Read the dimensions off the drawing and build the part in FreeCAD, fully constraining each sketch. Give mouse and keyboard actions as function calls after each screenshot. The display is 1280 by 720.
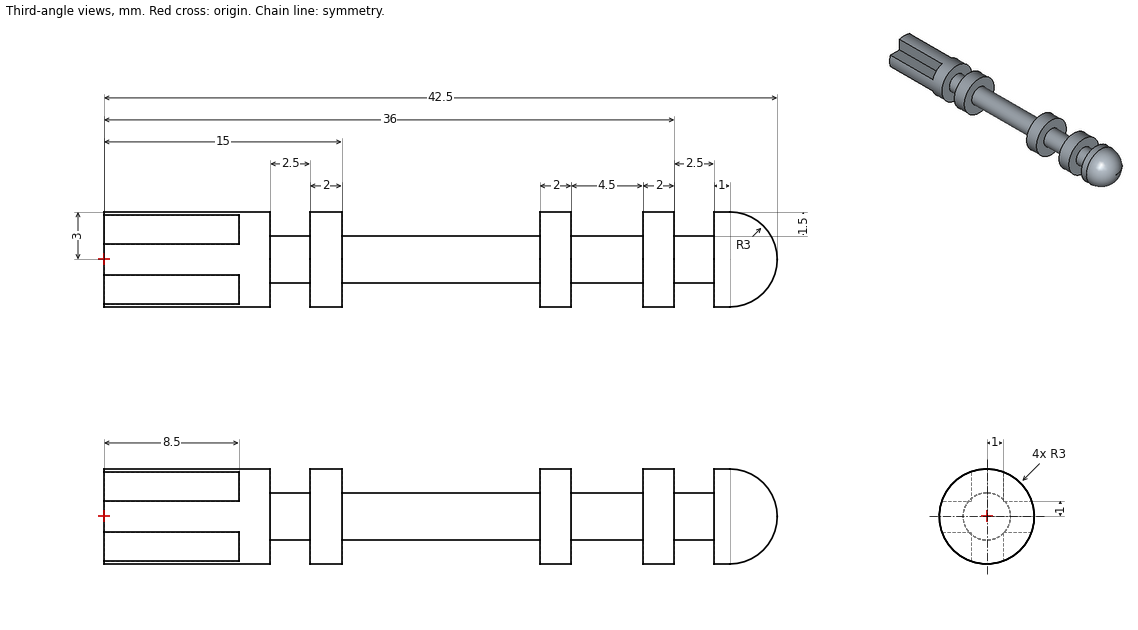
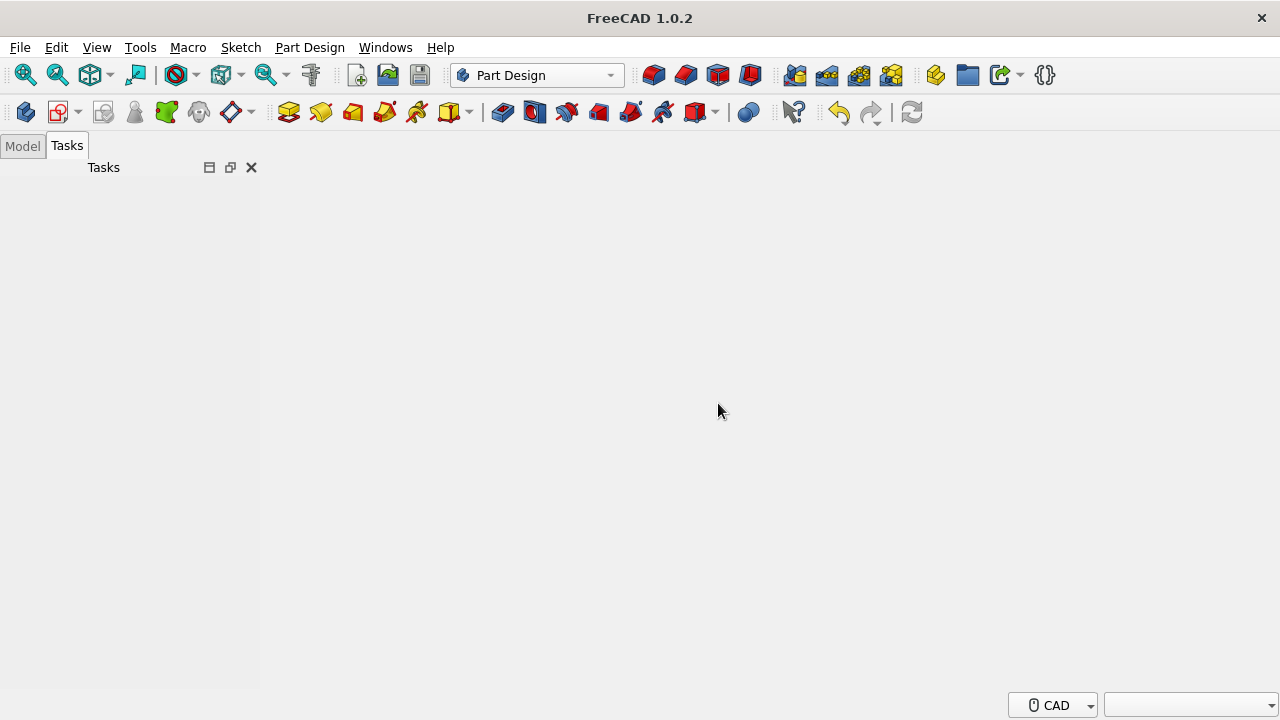
click(356, 76)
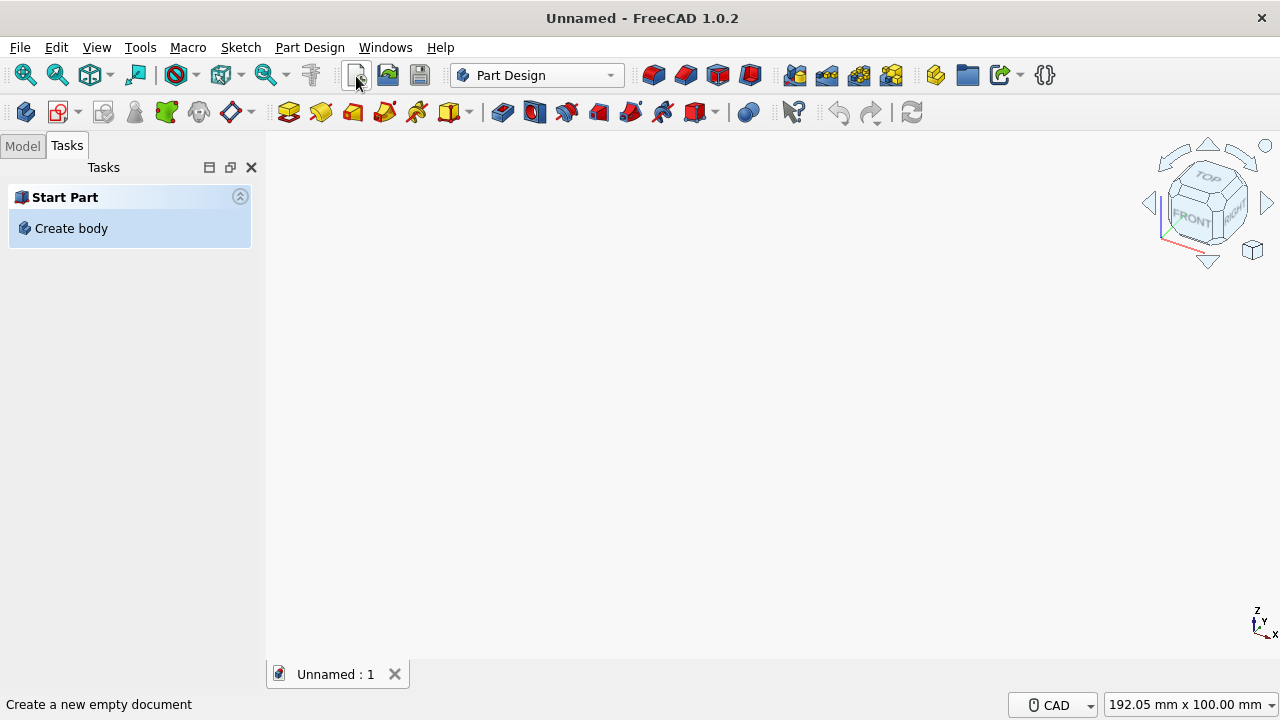
click(58, 112)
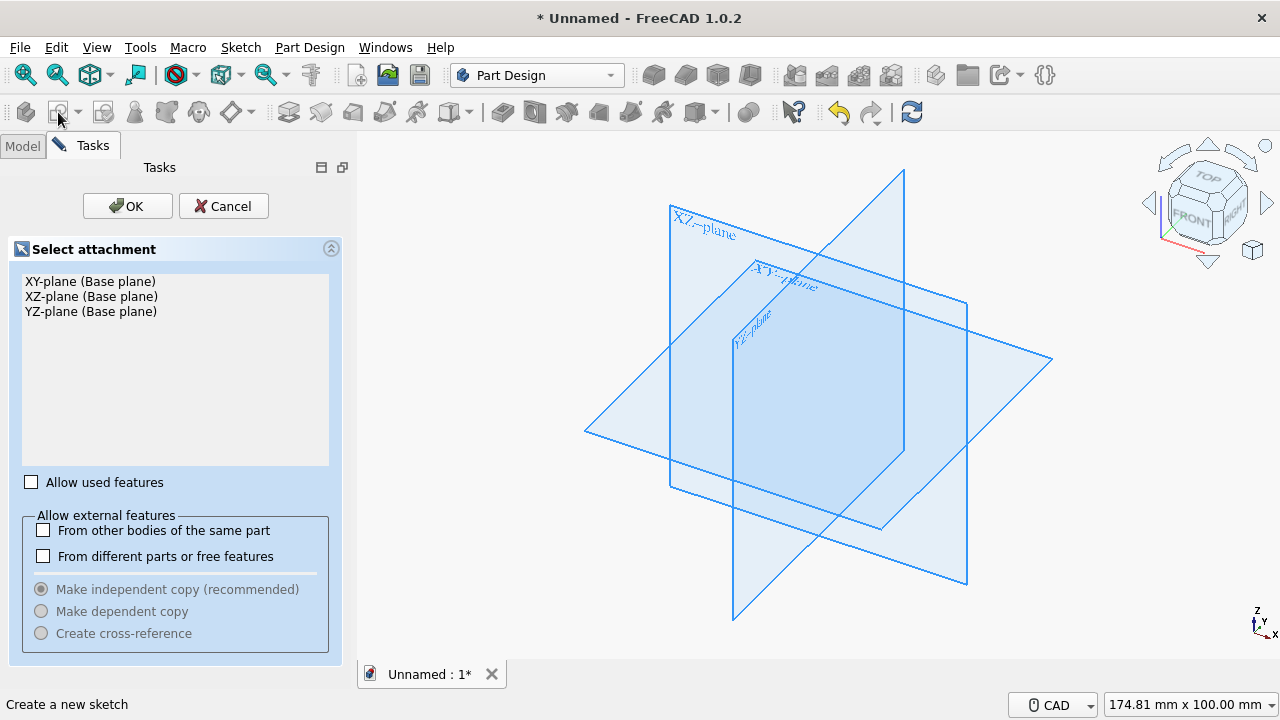
click(82, 282)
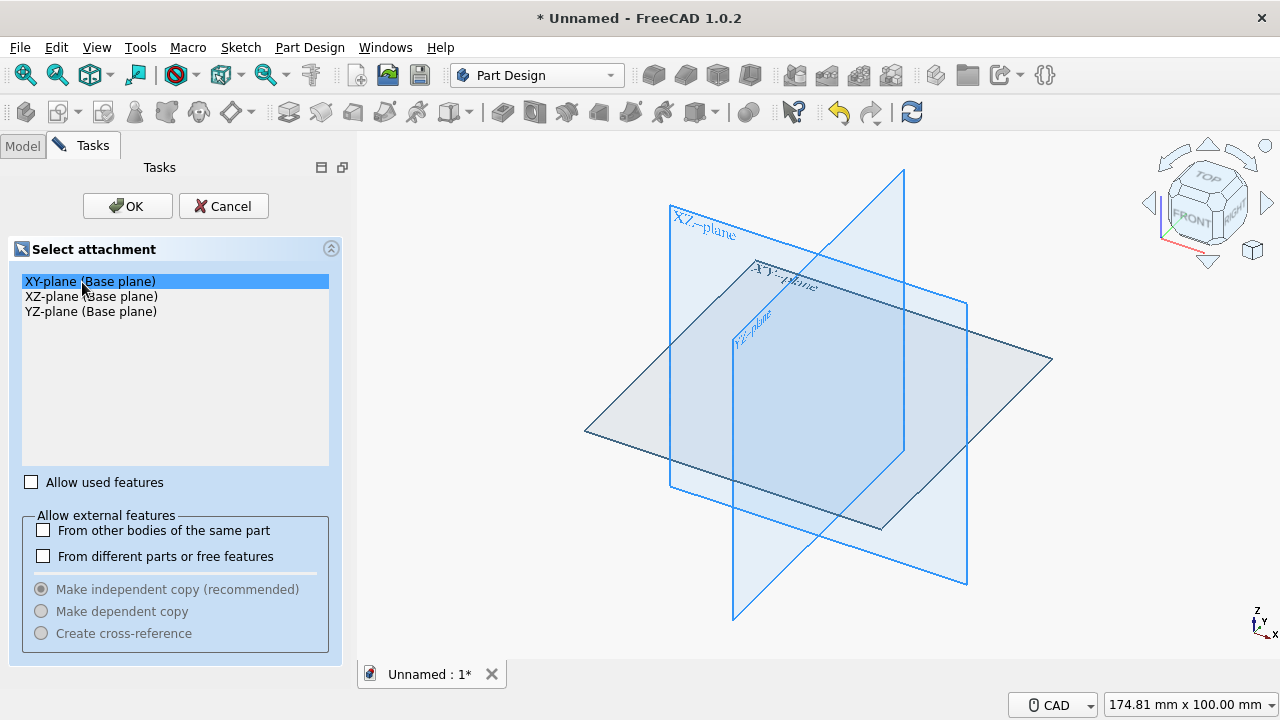
click(128, 206)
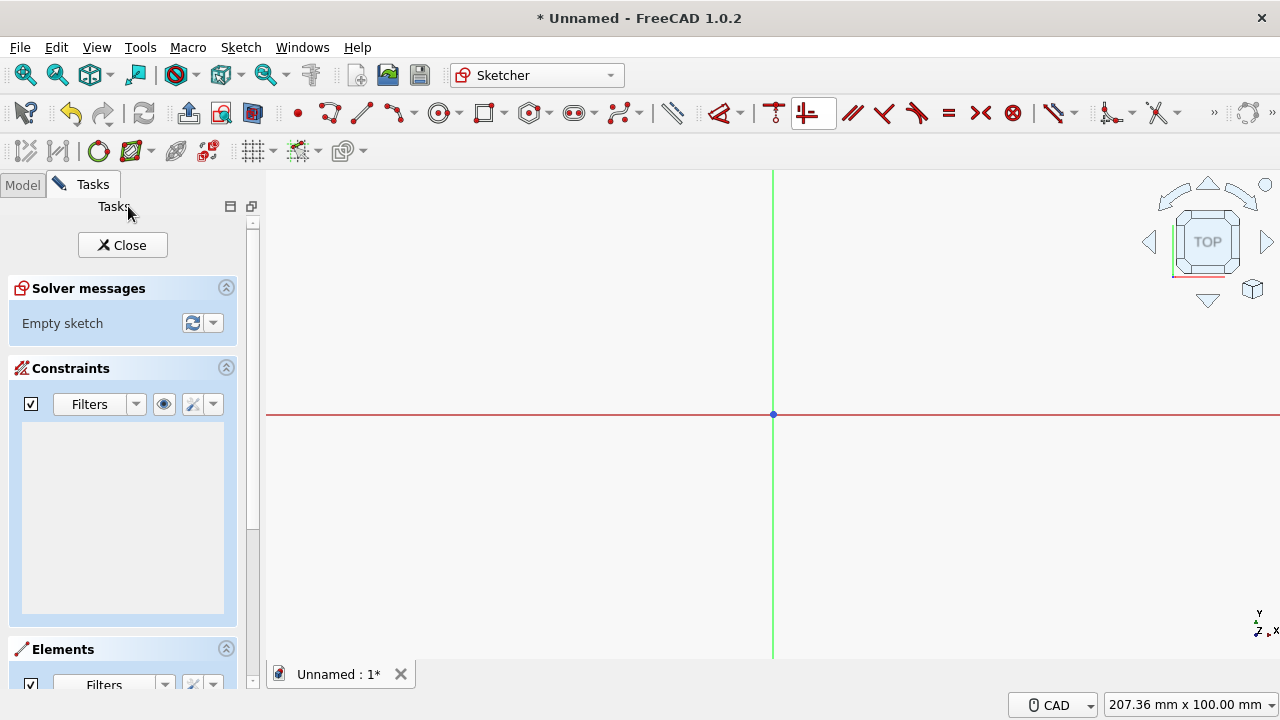
scroll(977, 403, up, 5)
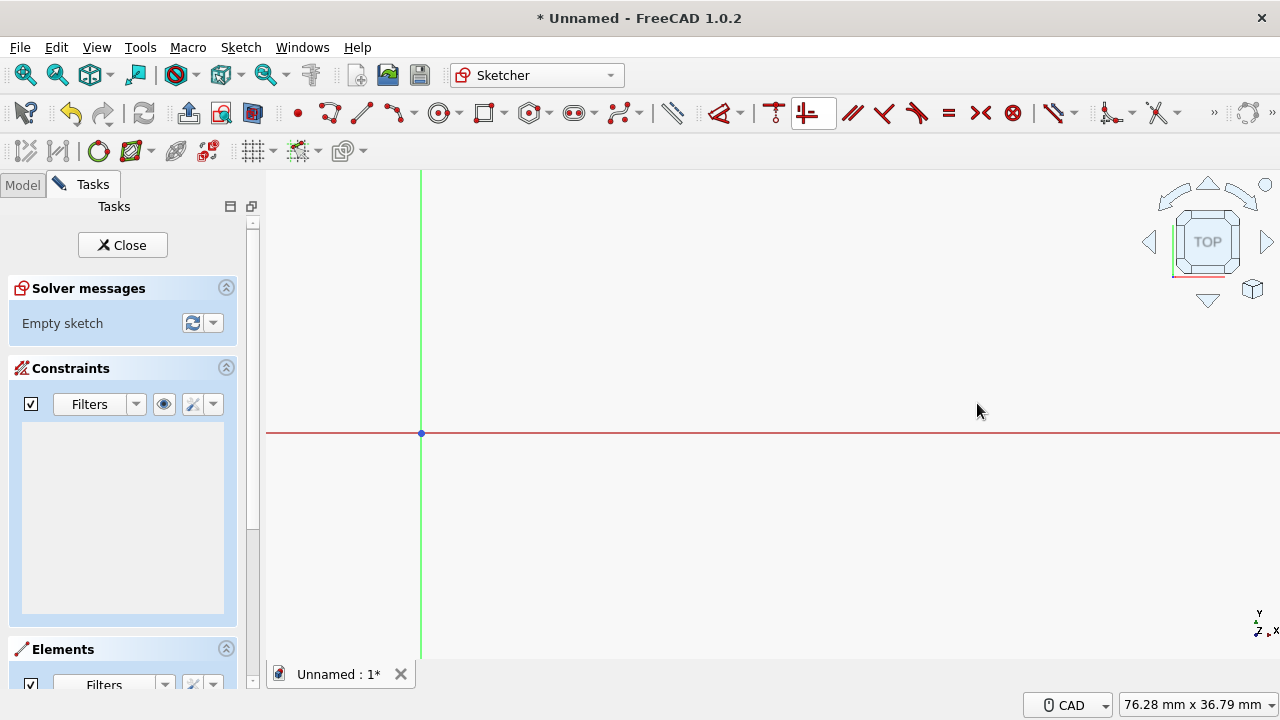
click(330, 114)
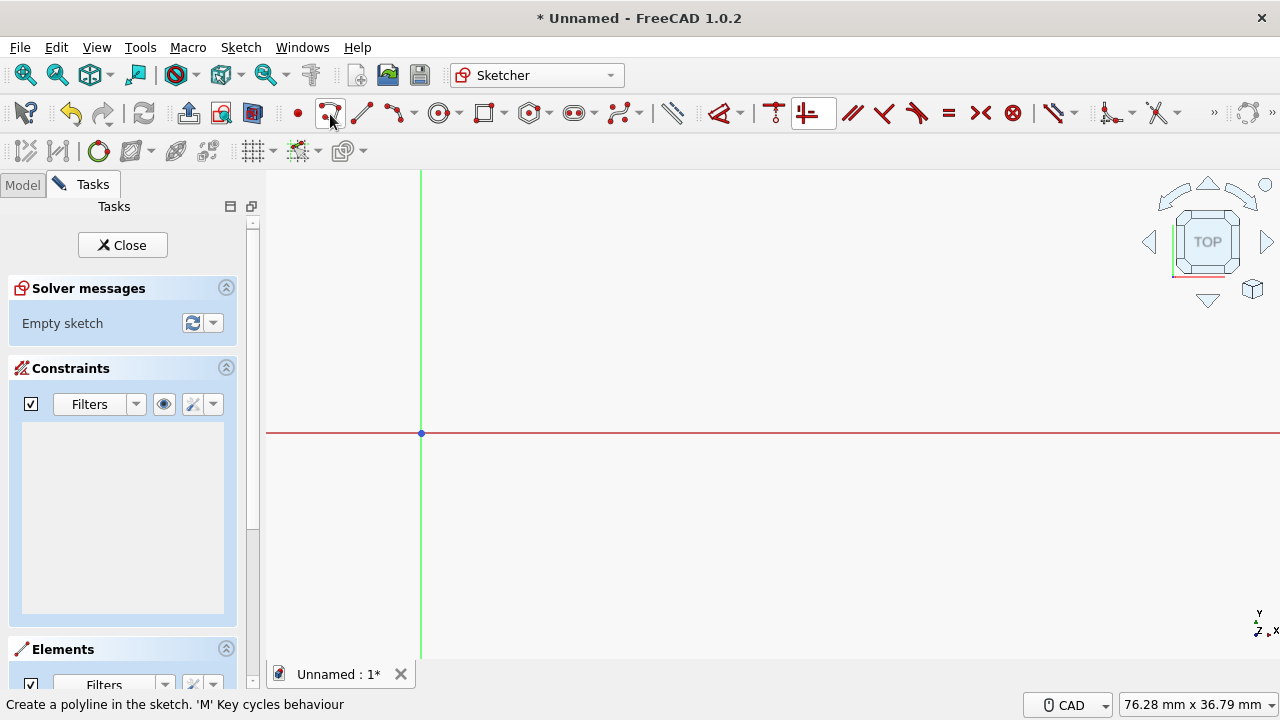
click(946, 394)
click(933, 394)
click(933, 414)
click(900, 414)
click(900, 394)
click(873, 394)
click(873, 414)
click(813, 414)
click(813, 394)
click(787, 394)
click(787, 414)
click(621, 414)
click(621, 394)
click(594, 394)
click(594, 414)
click(561, 414)
click(561, 394)
click(421, 394)
click(421, 433)
click(986, 424)
right_click(986, 424)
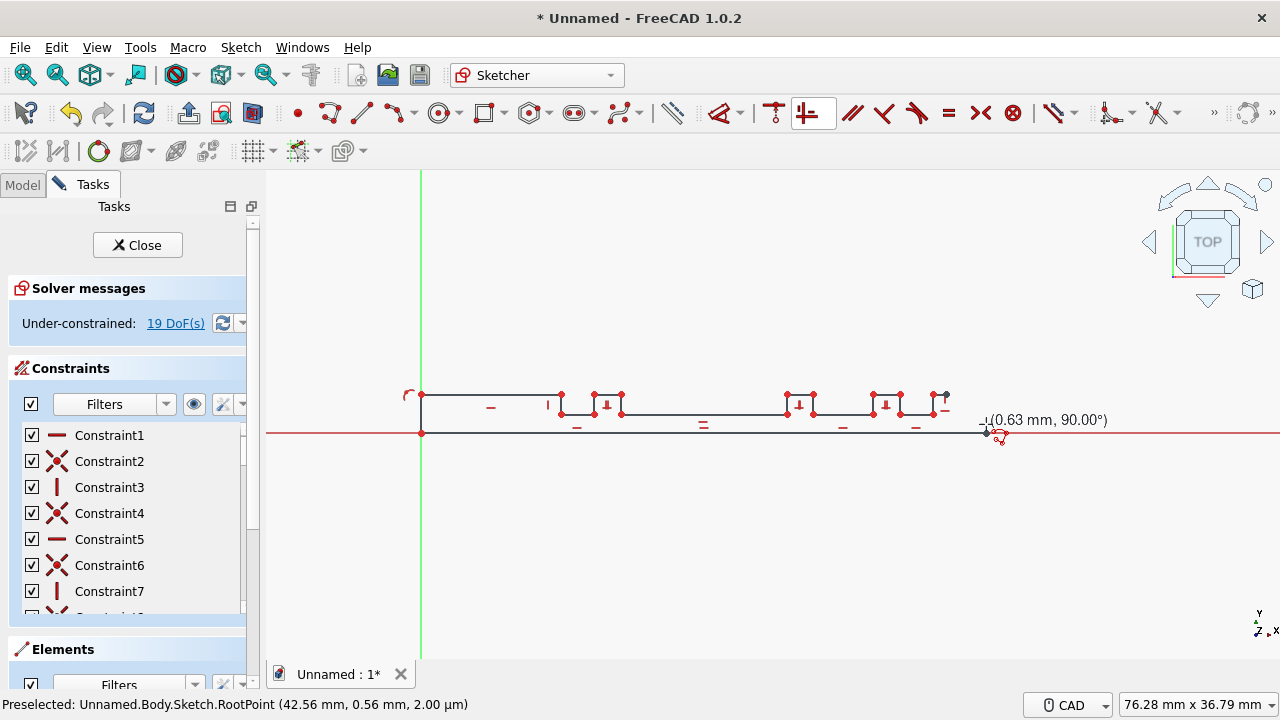
click(394, 114)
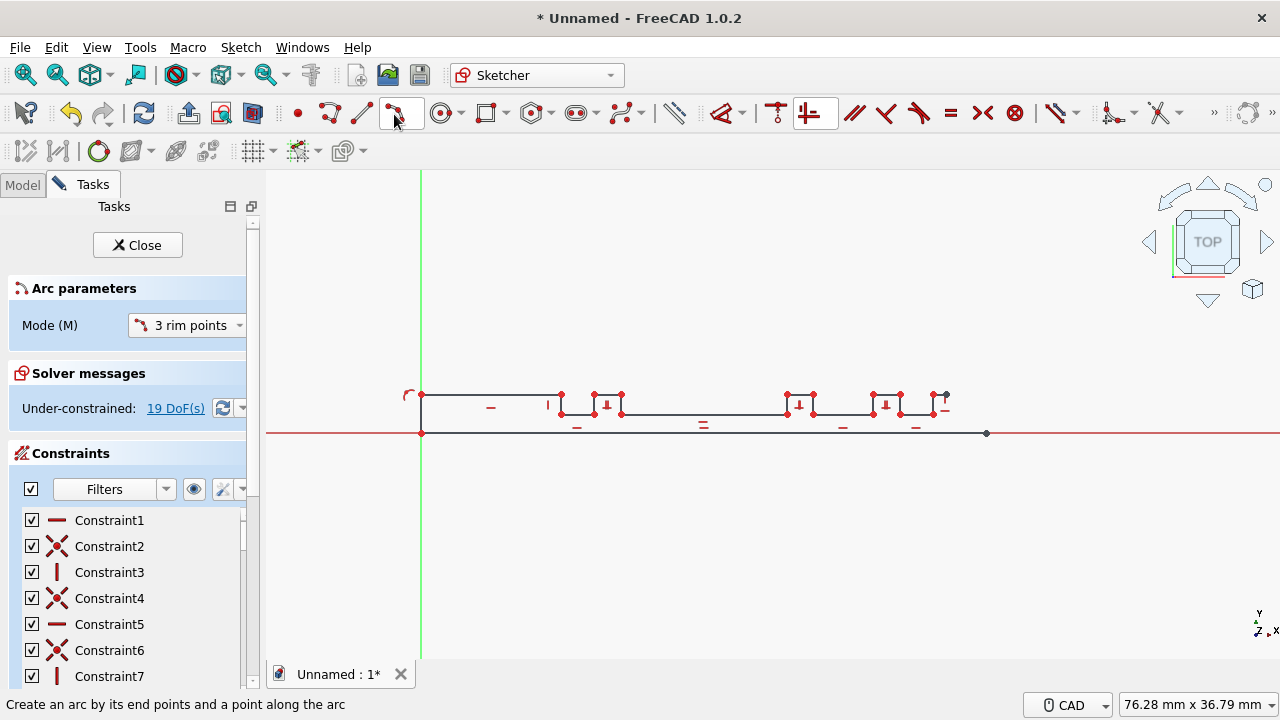
click(986, 424)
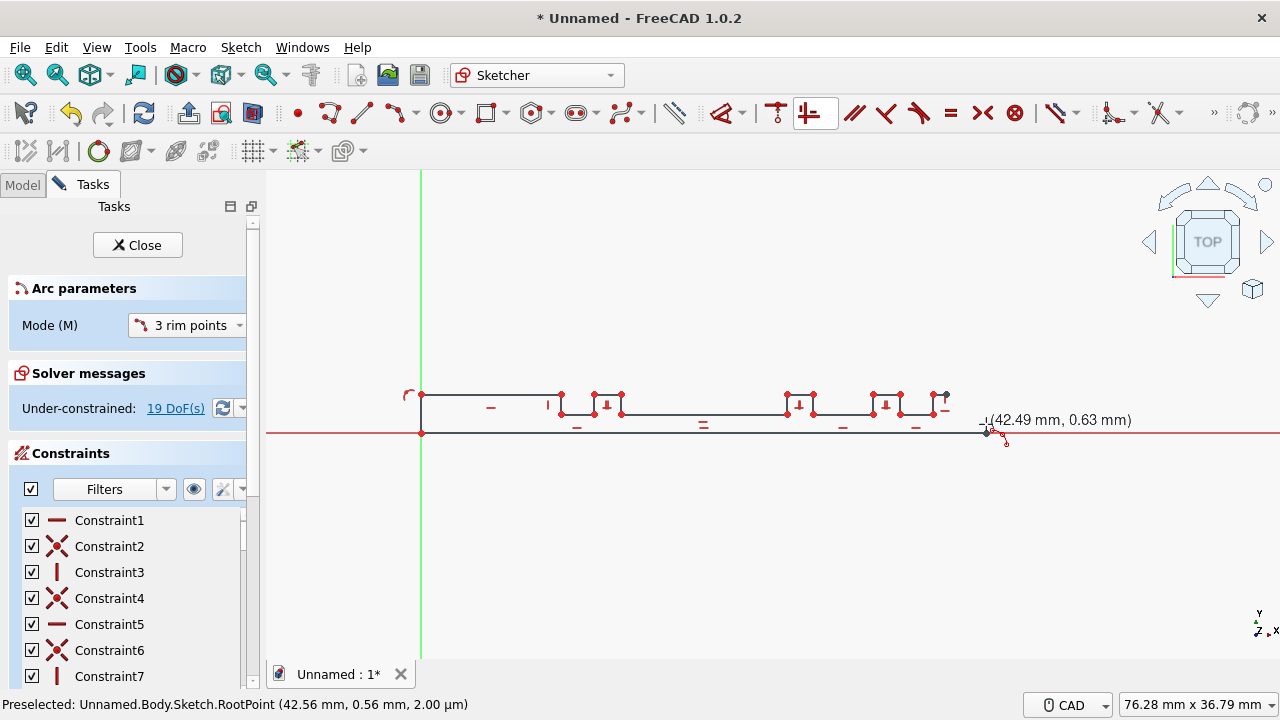
scroll(946, 394, up, 5)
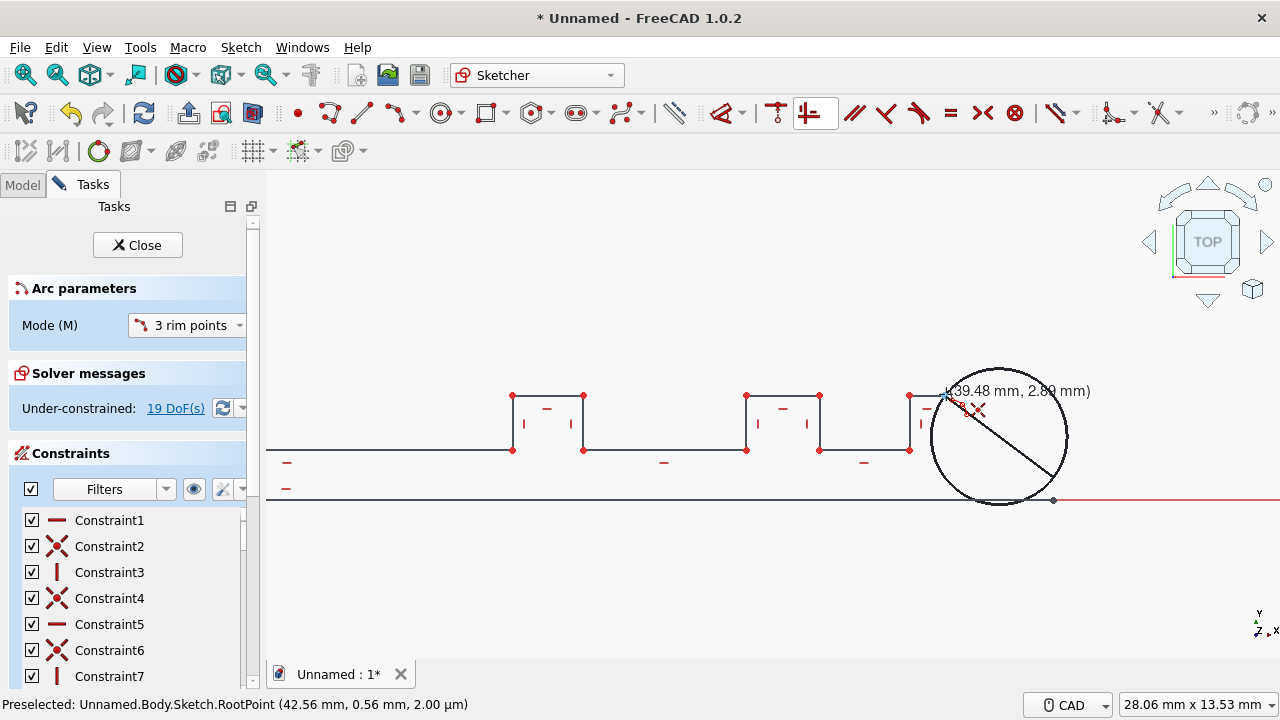
click(945, 396)
click(1022, 424)
key(Escape)